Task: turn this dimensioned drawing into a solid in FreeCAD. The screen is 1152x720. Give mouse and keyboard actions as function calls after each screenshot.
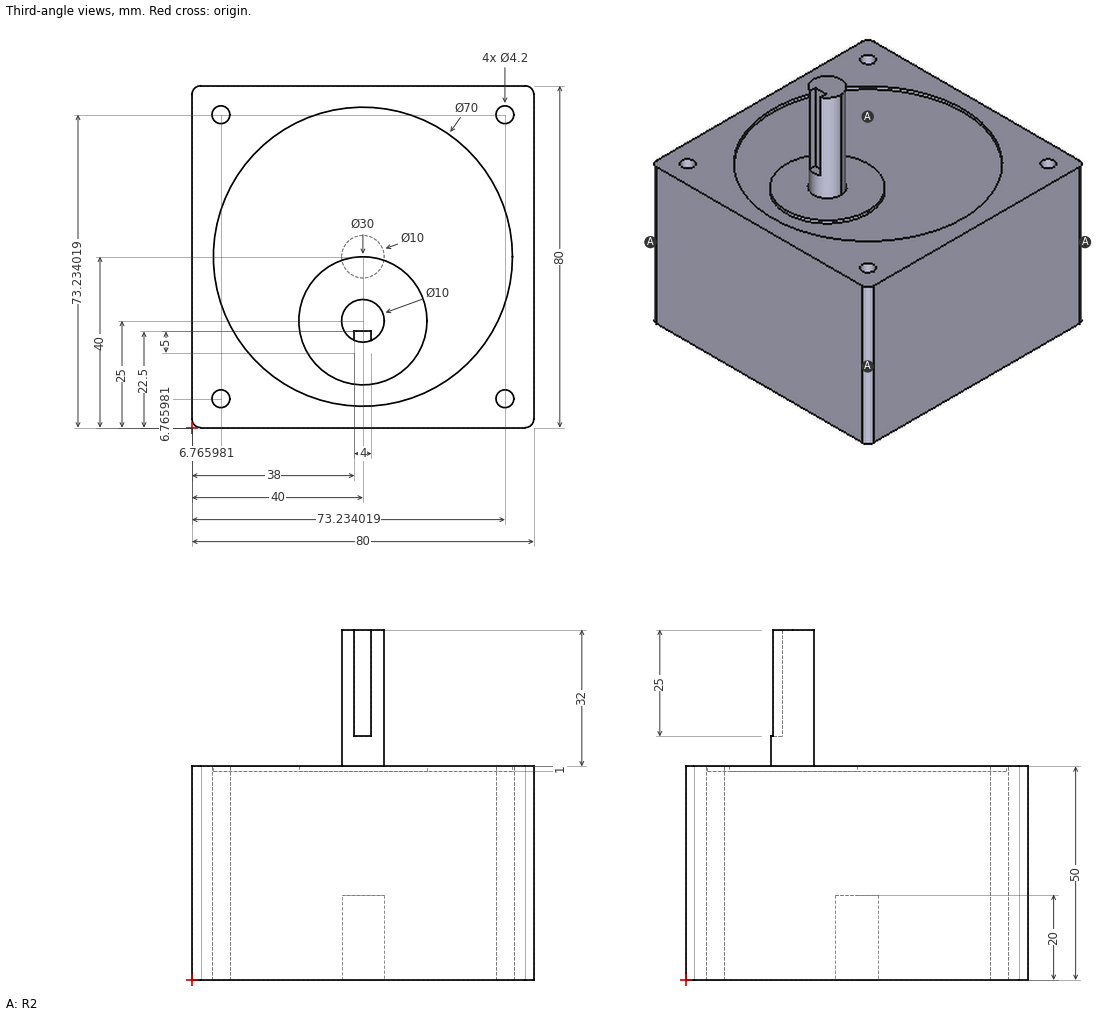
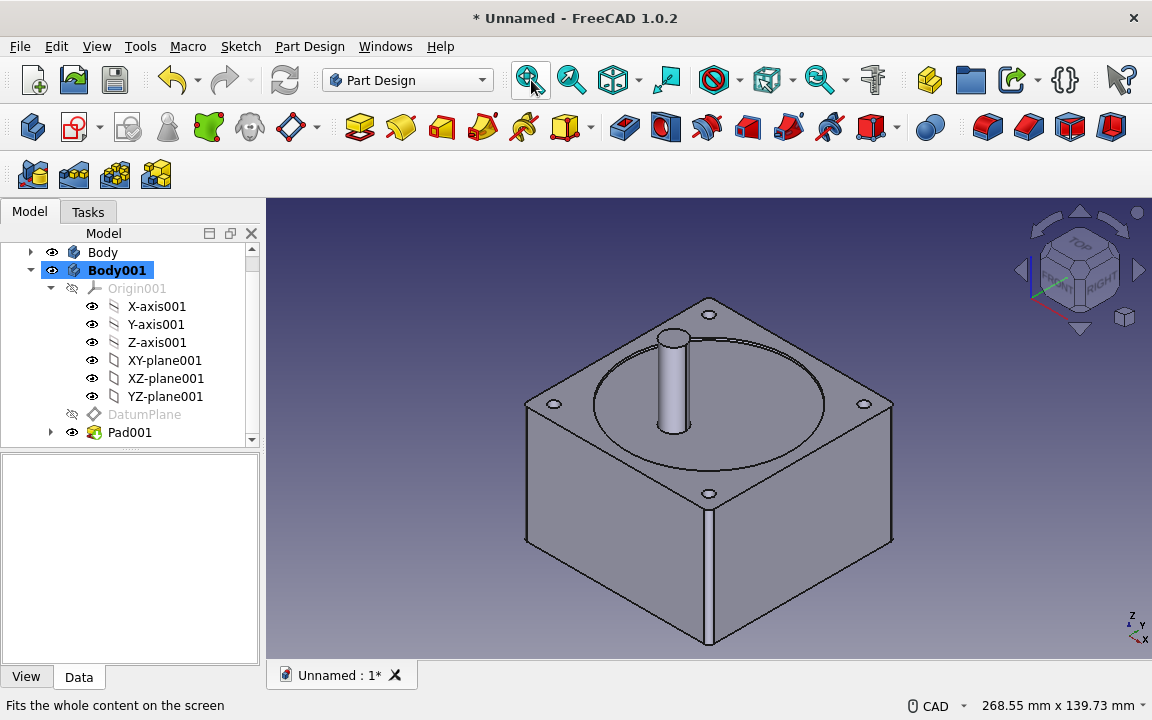
click(531, 80)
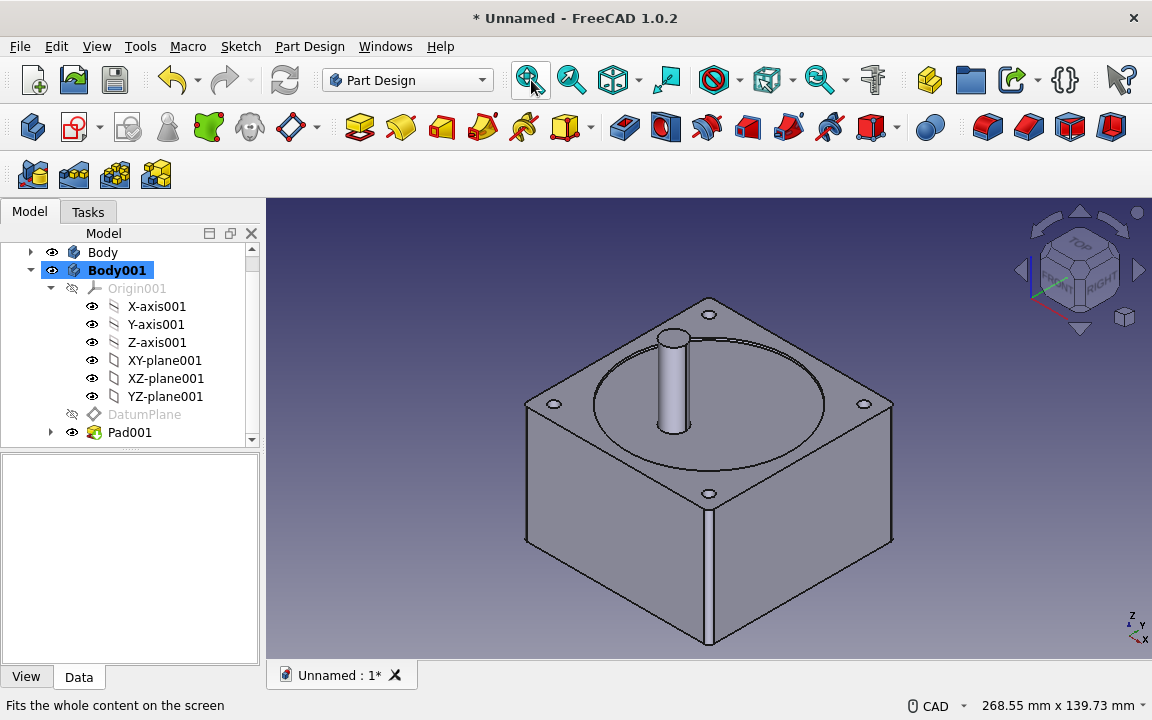
click(674, 337)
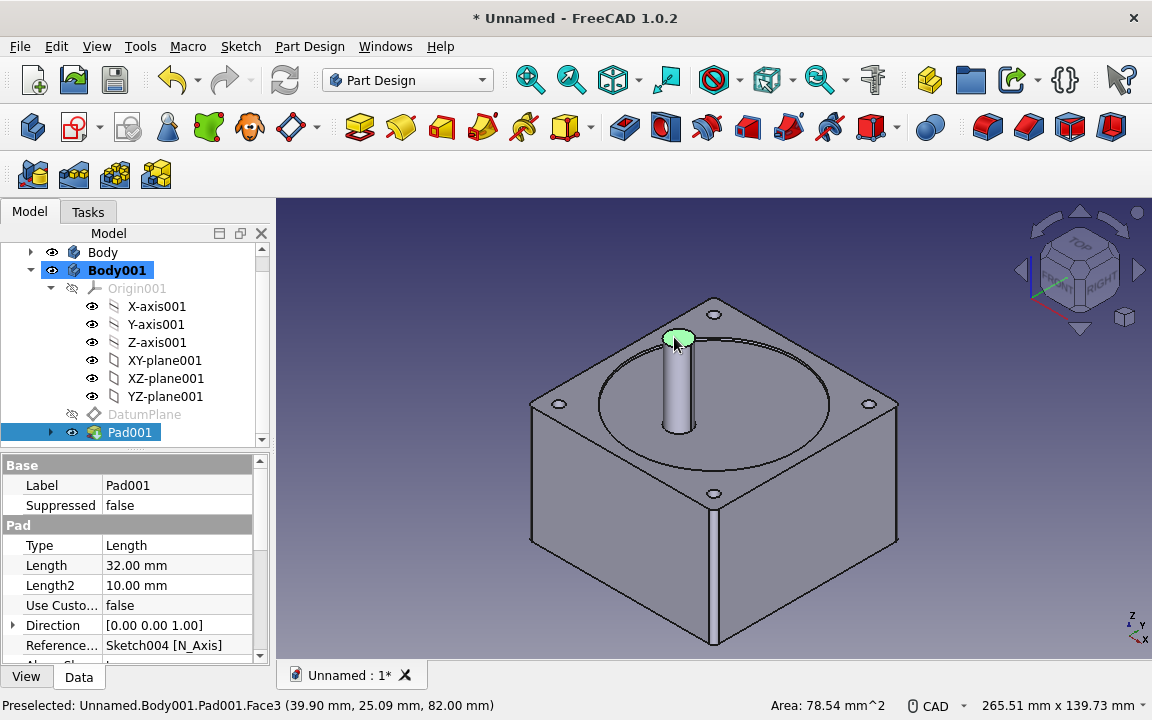
click(74, 128)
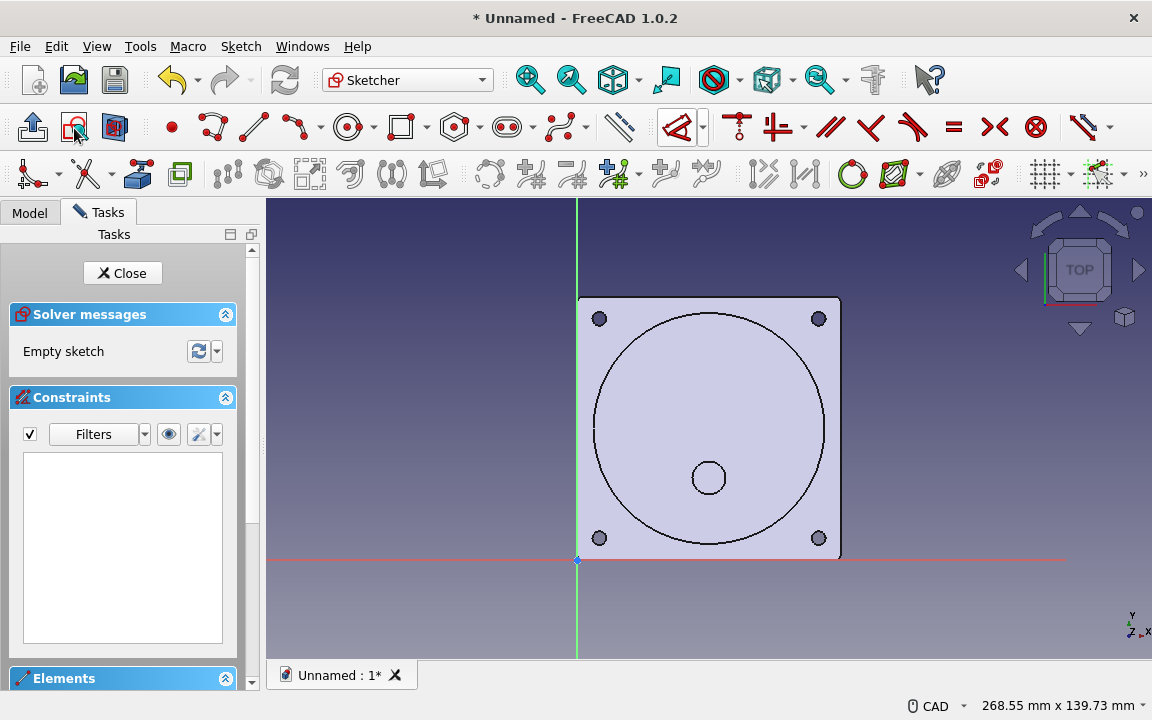
scroll(713, 499, up, 14)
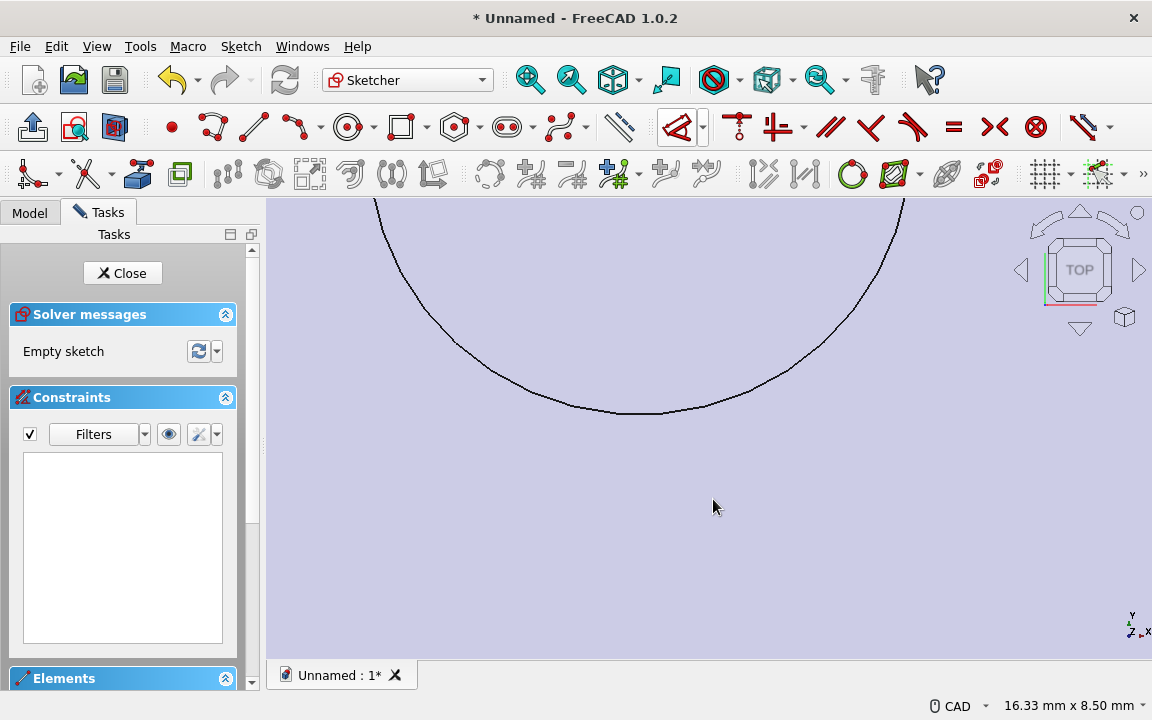
key(g)
key(r)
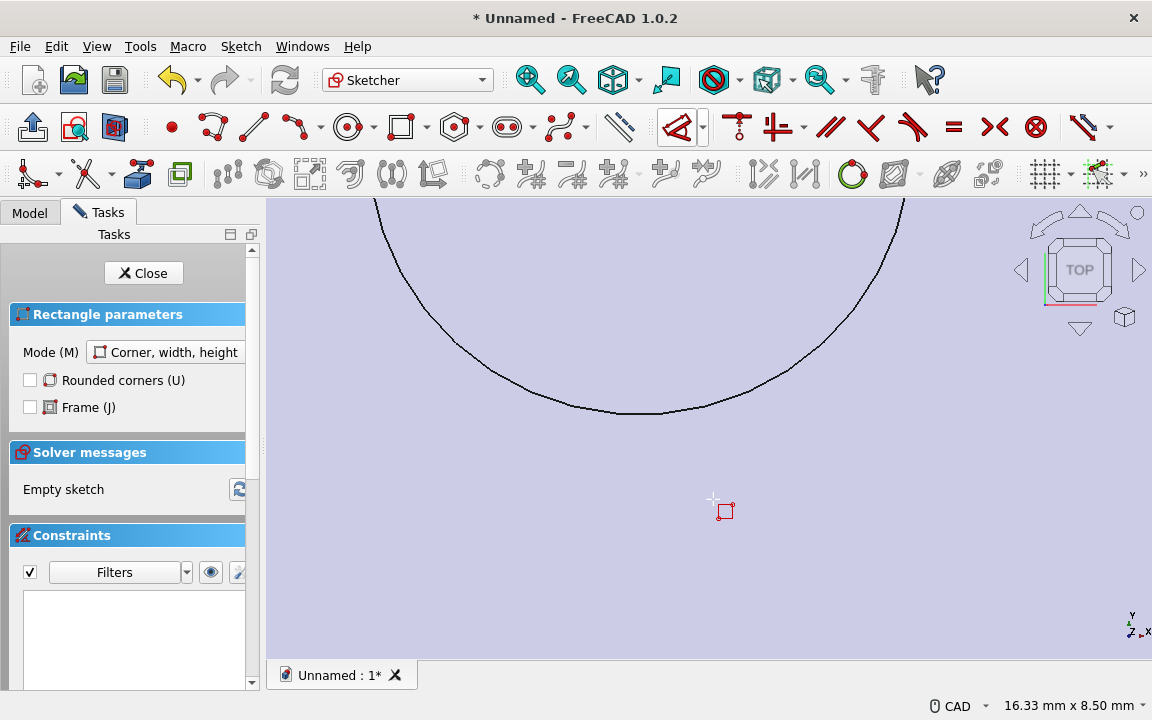
click(531, 279)
click(748, 550)
key(Escape)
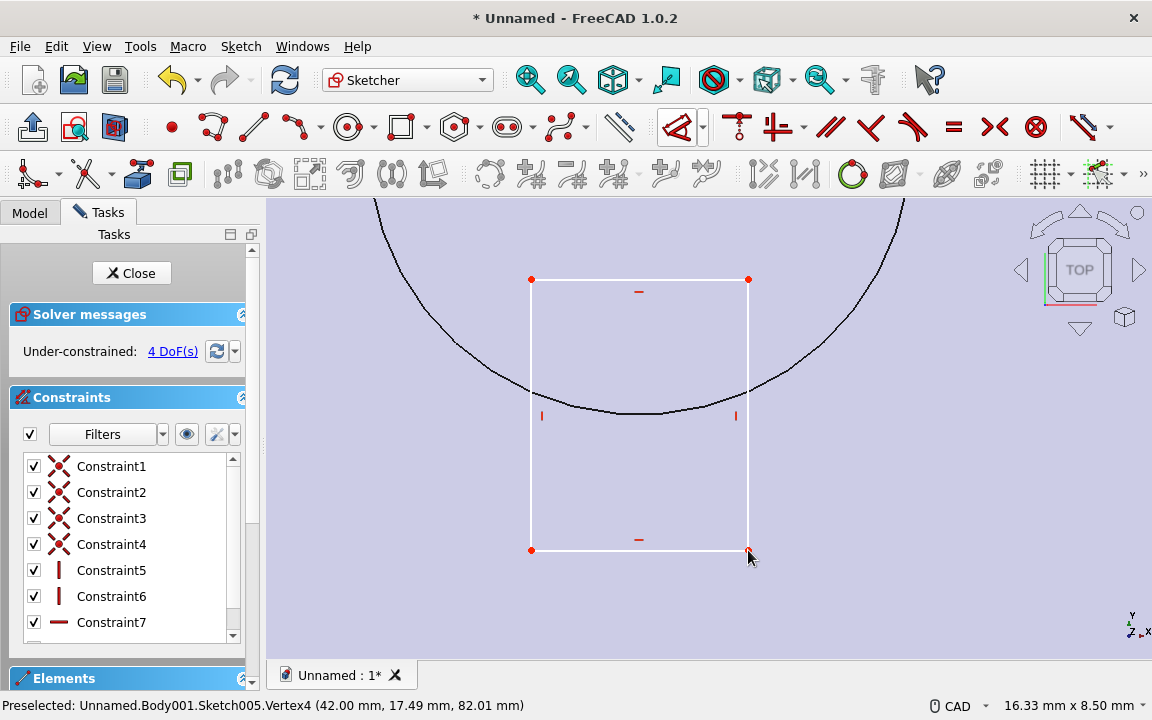
click(531, 361)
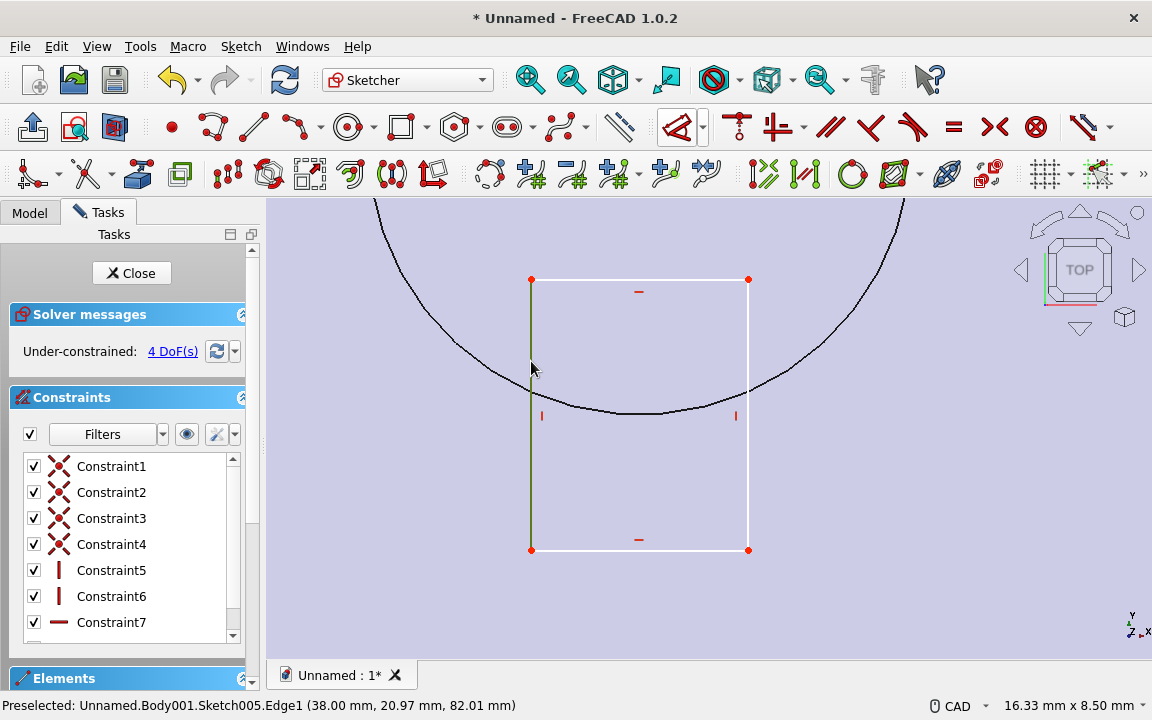
key(i)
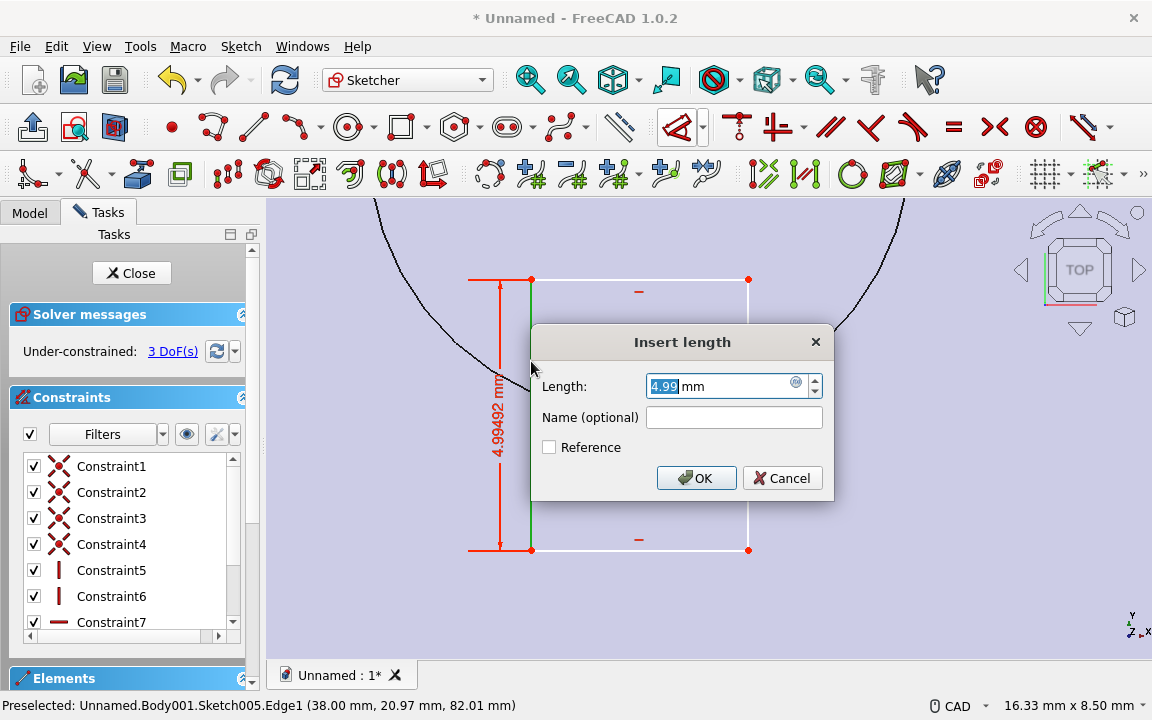
text(5)
key(Return)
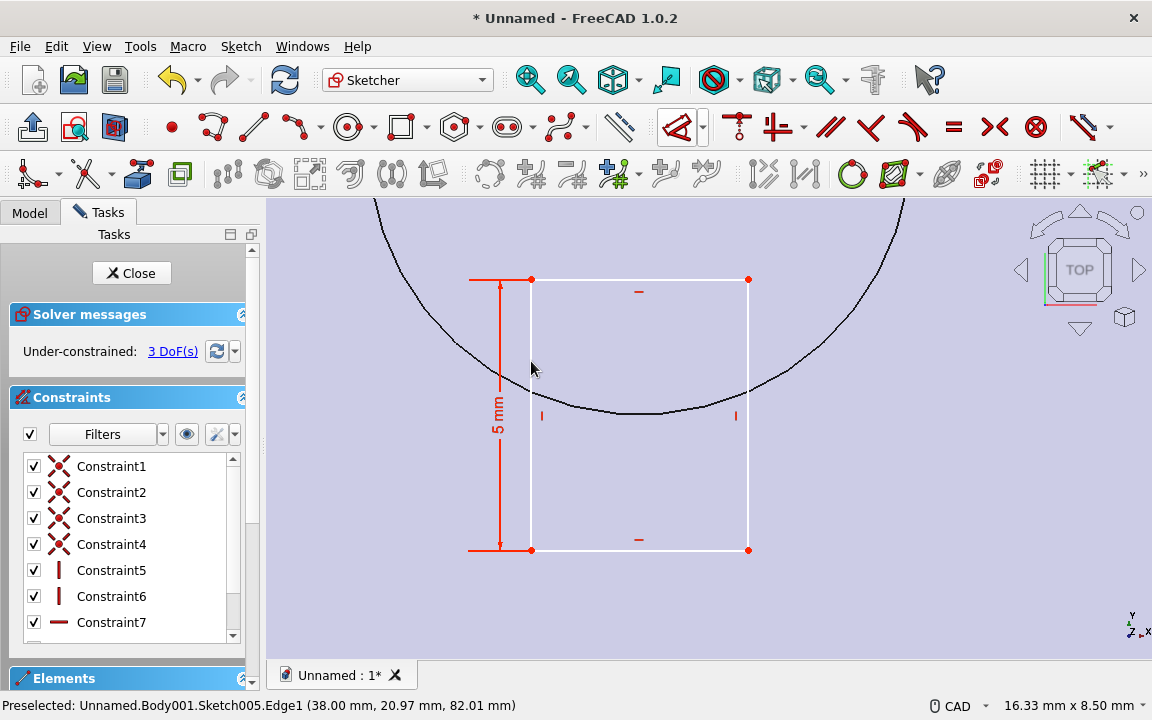
click(596, 551)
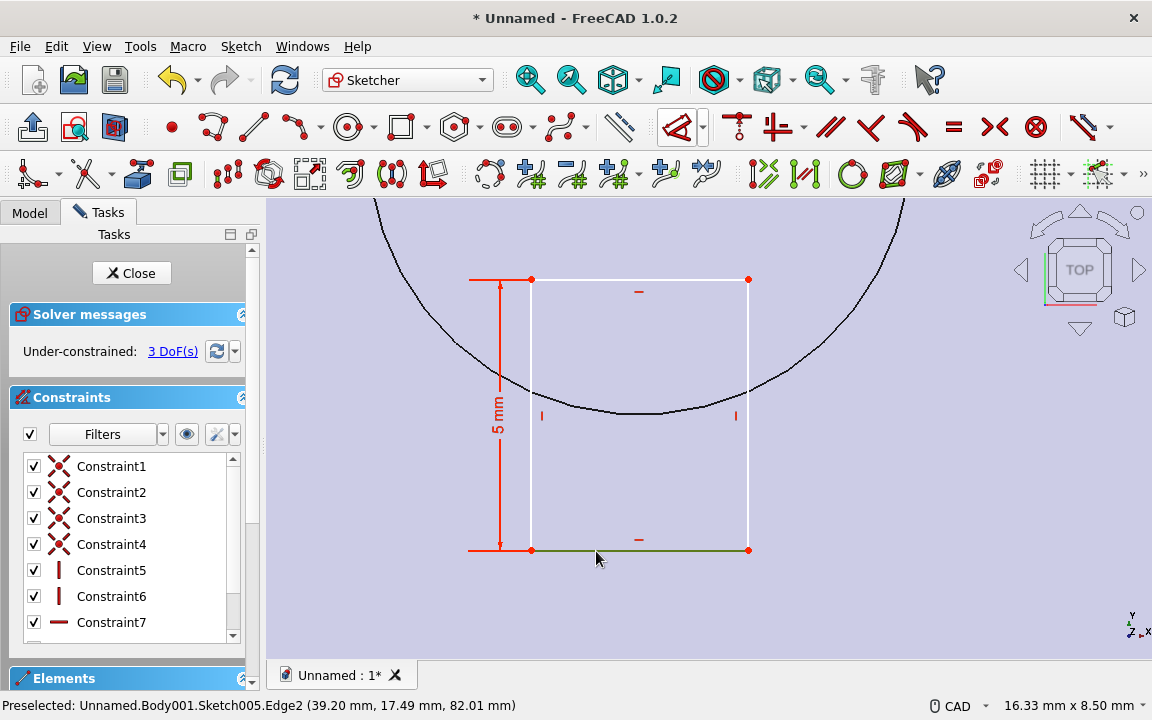
key(l)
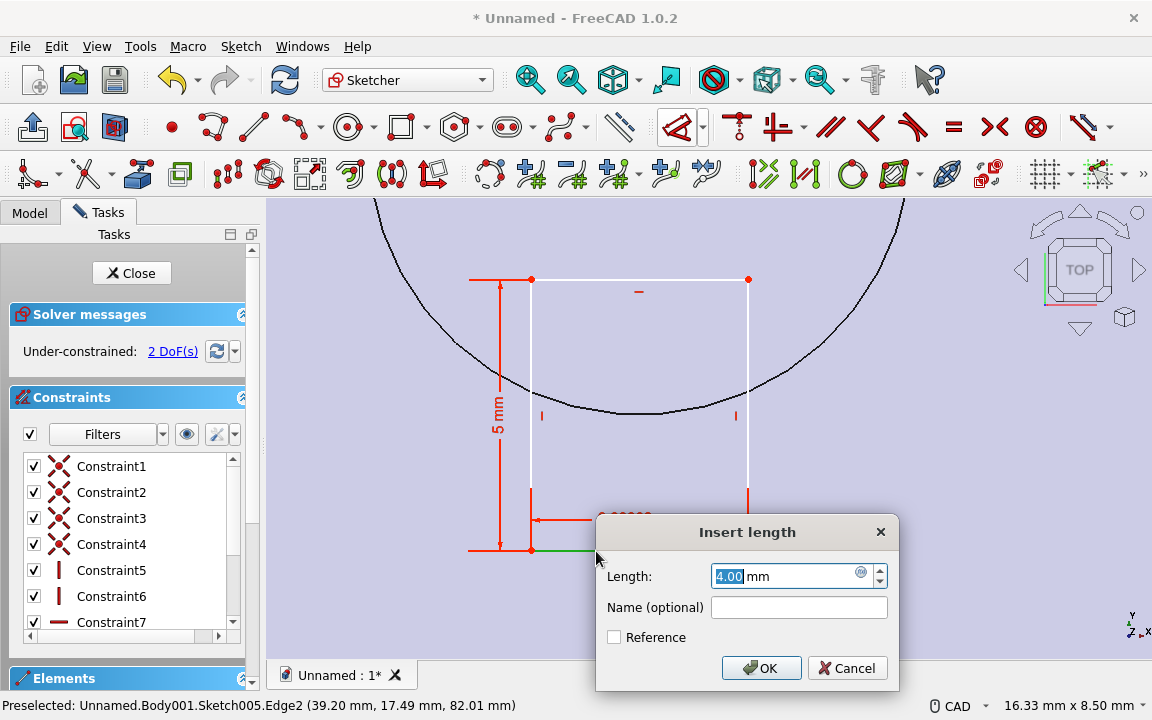
text(4)
key(Return)